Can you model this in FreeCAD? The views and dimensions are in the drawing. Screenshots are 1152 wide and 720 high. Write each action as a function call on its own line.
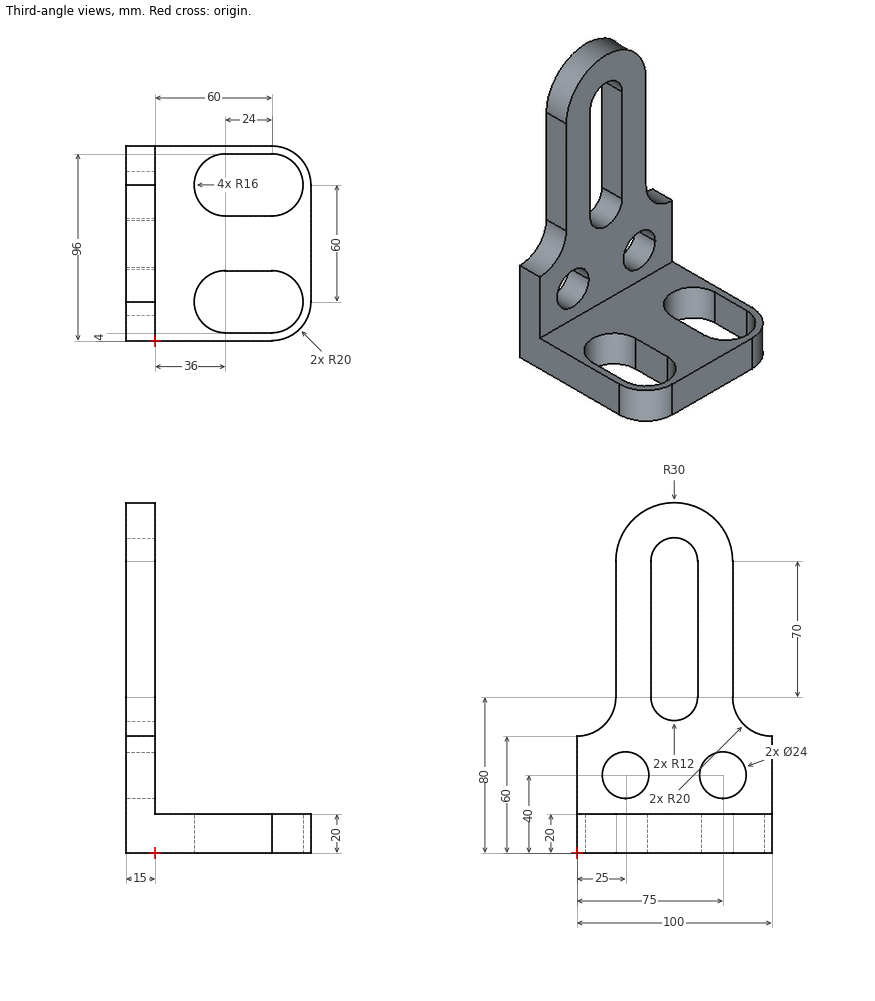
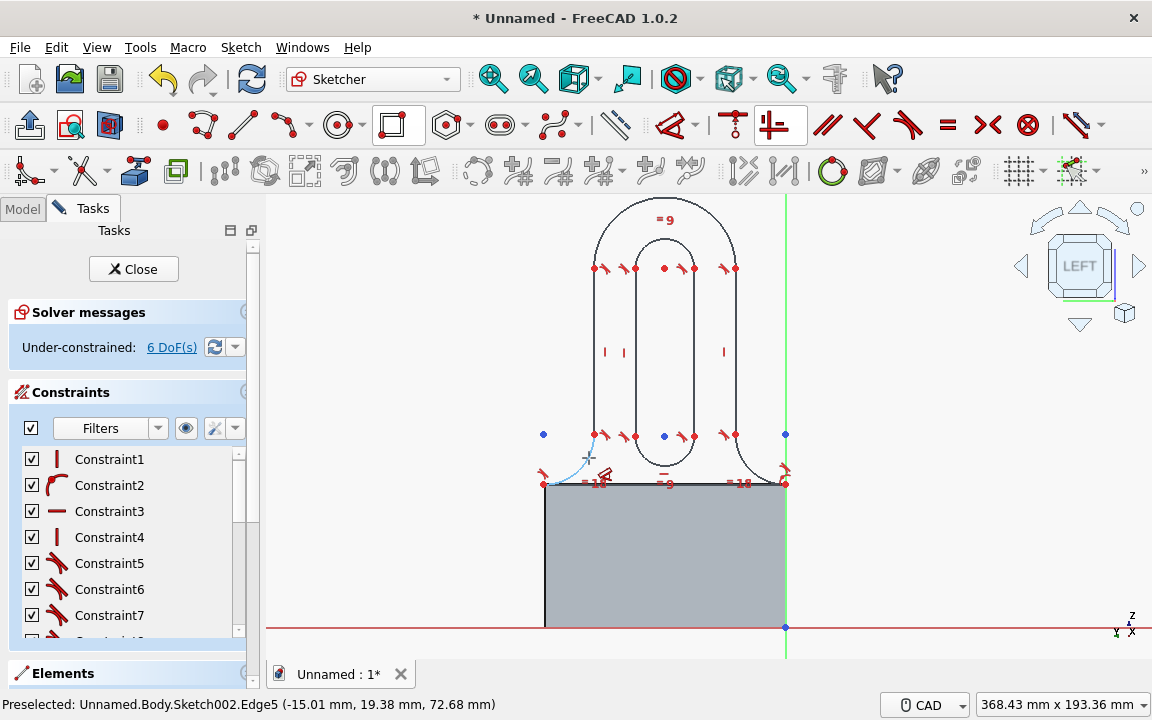
click(589, 457)
click(618, 471)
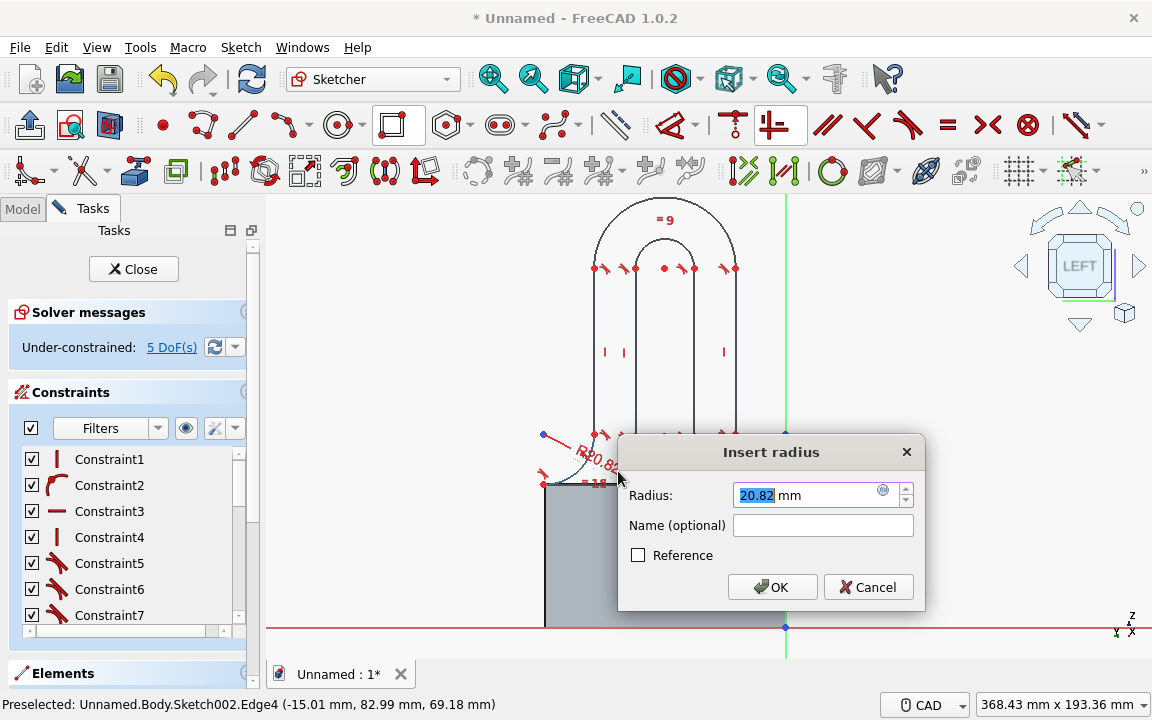
text(20)
key(Return)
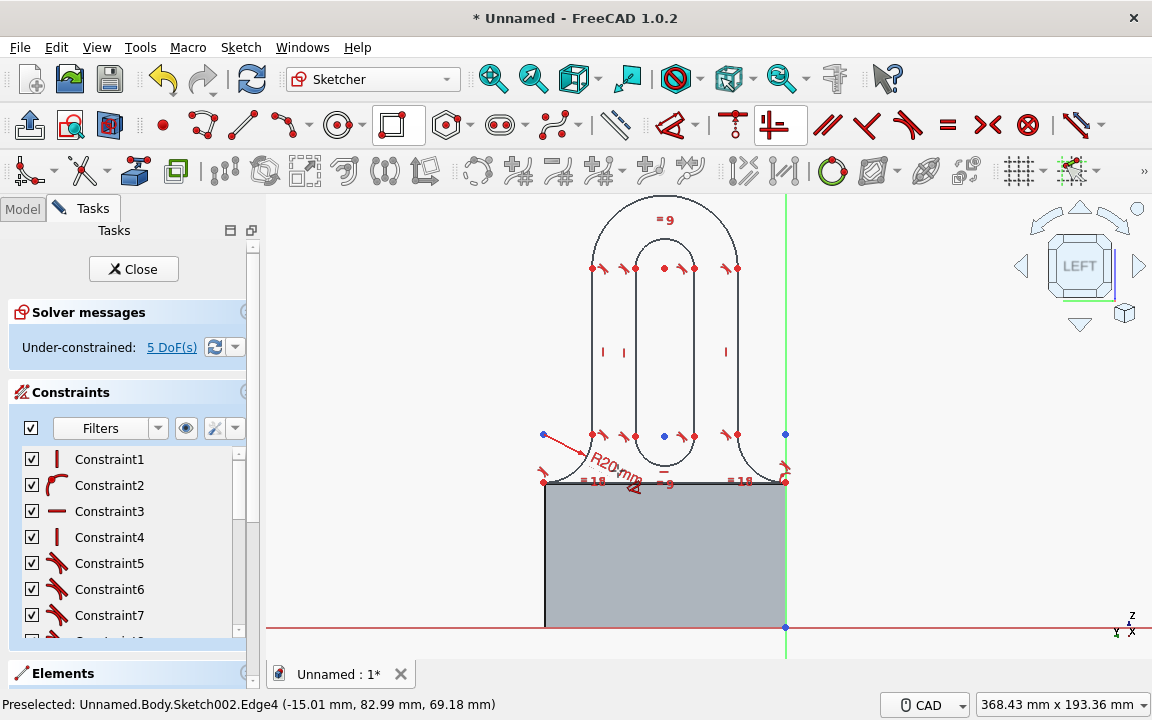
click(724, 226)
click(769, 256)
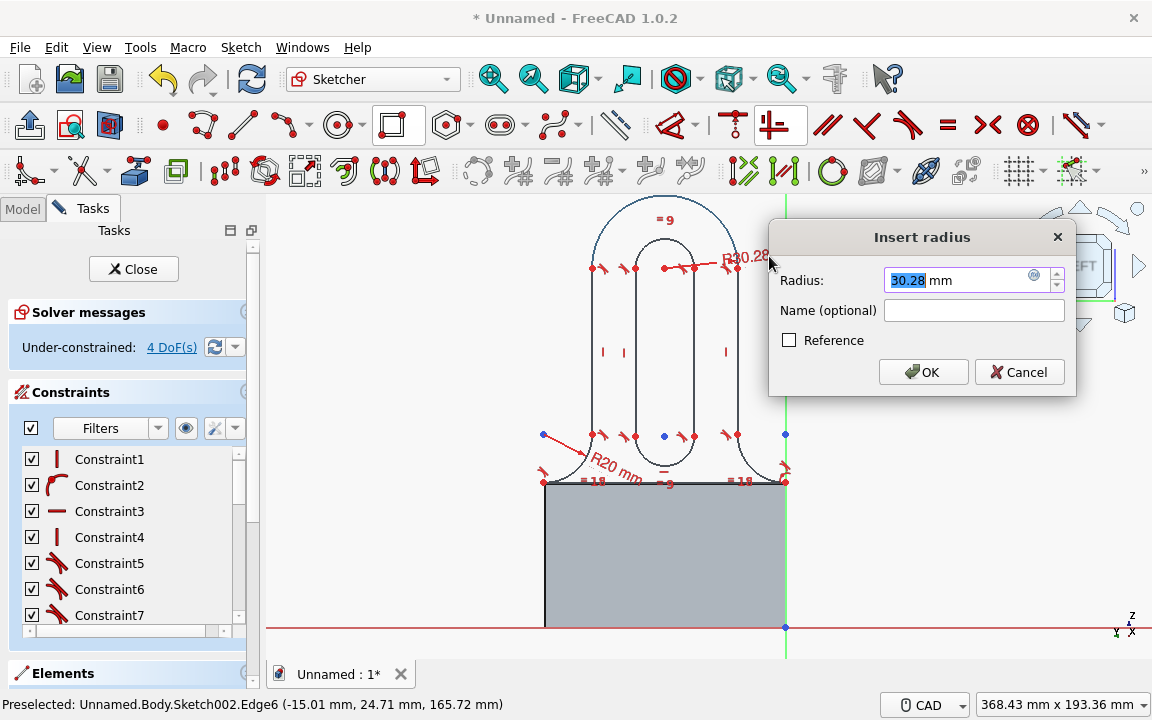
text(30)
key(Return)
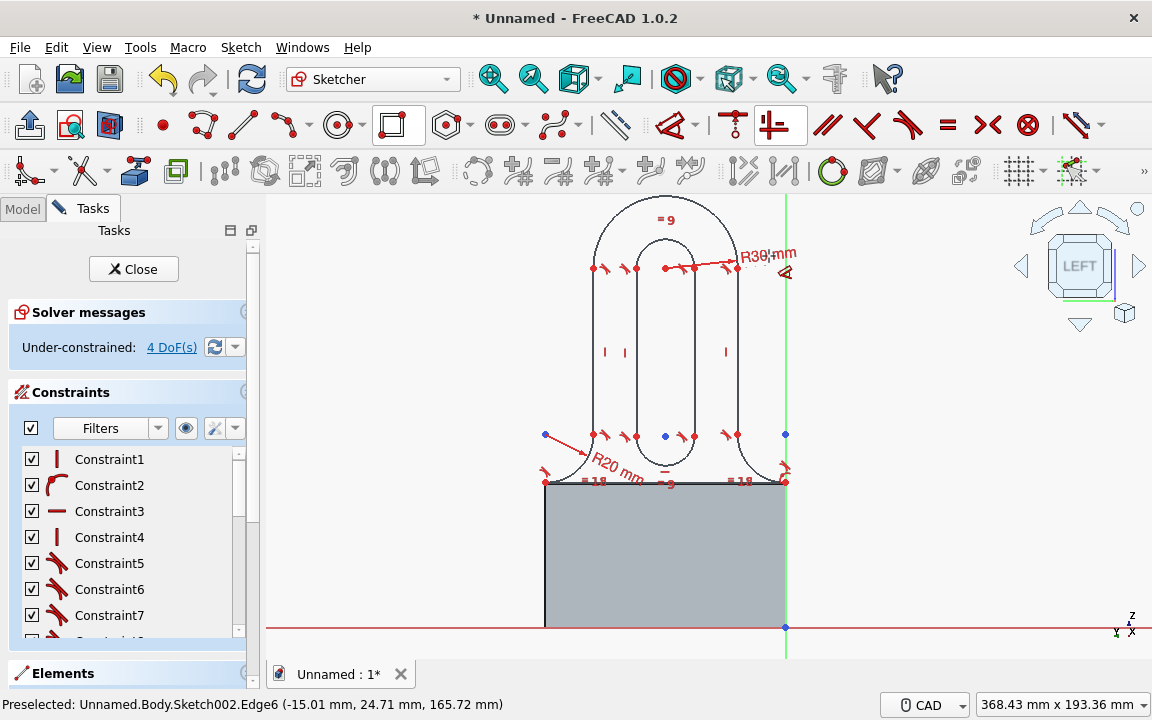
scroll(649, 460, up, 2)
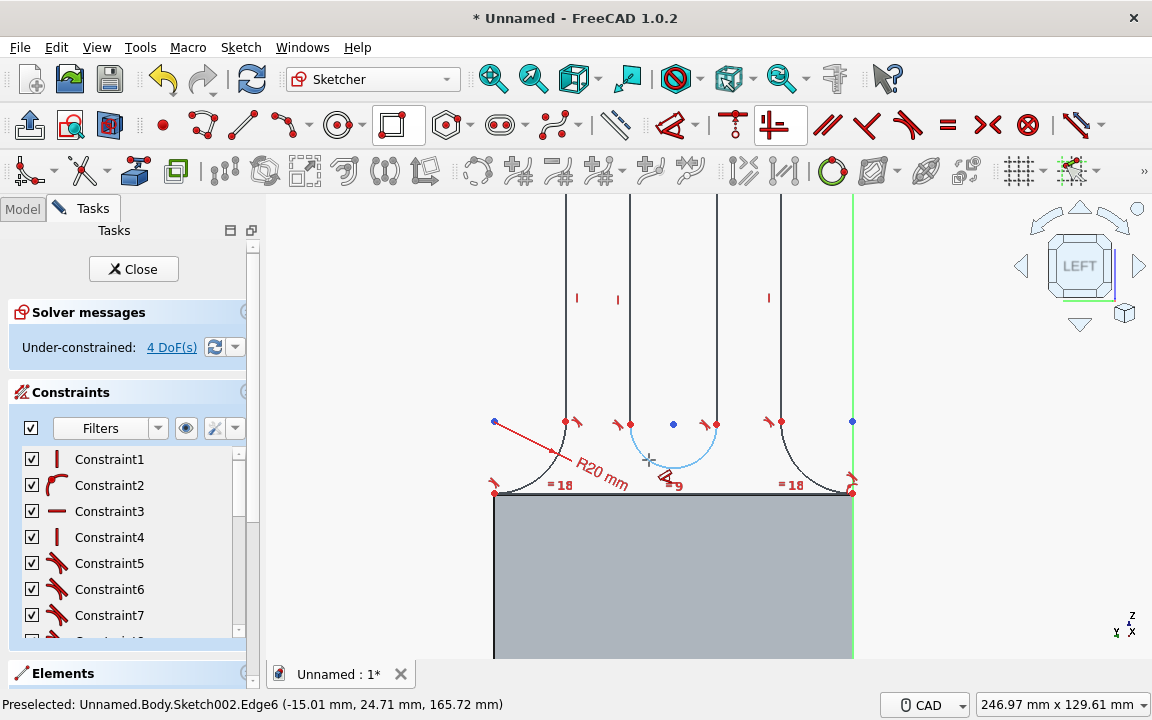
click(648, 460)
click(598, 421)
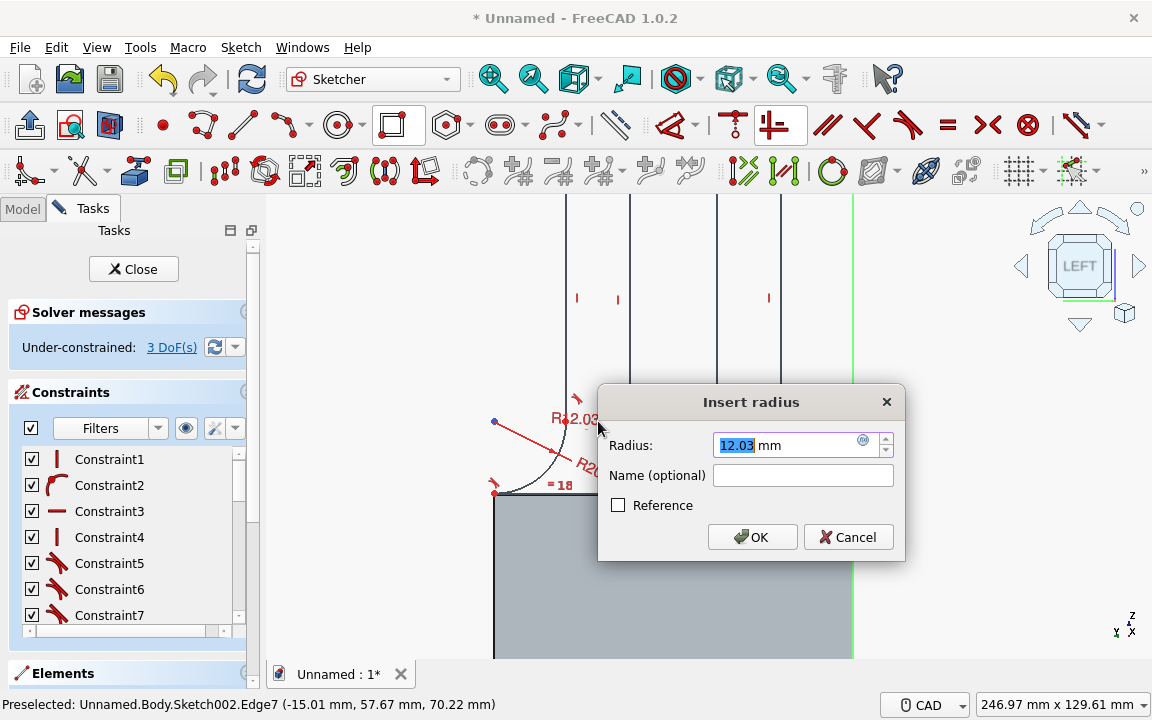
text(12)
key(Return)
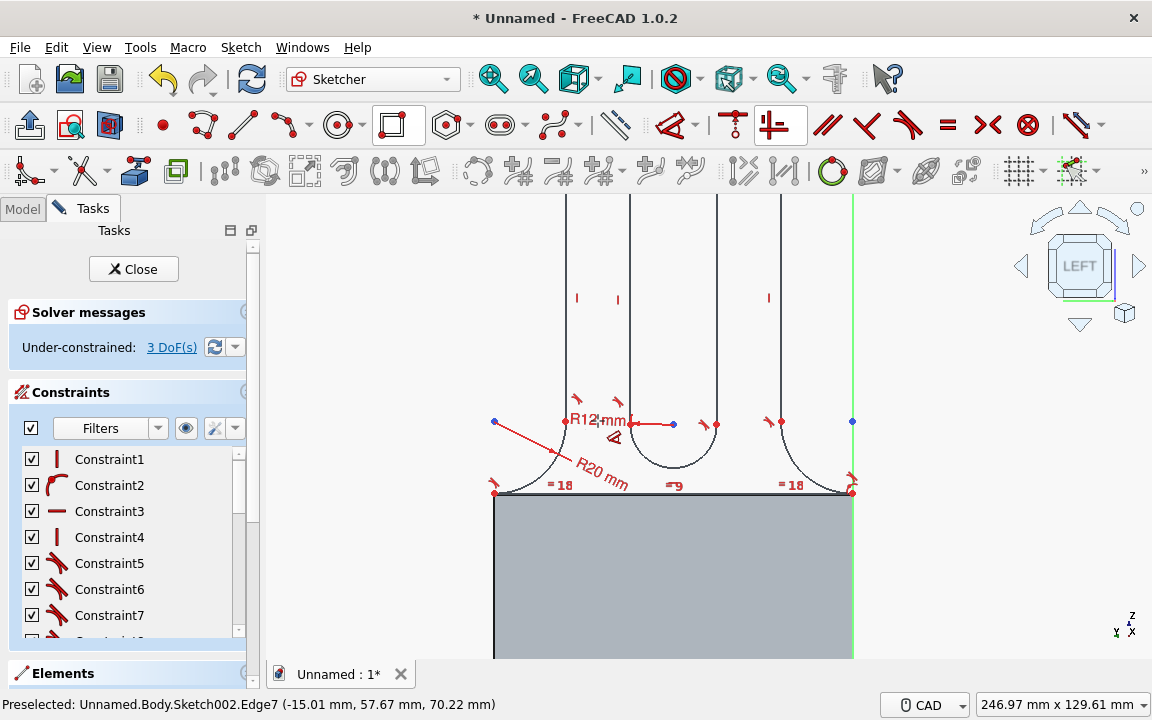
click(566, 248)
click(532, 322)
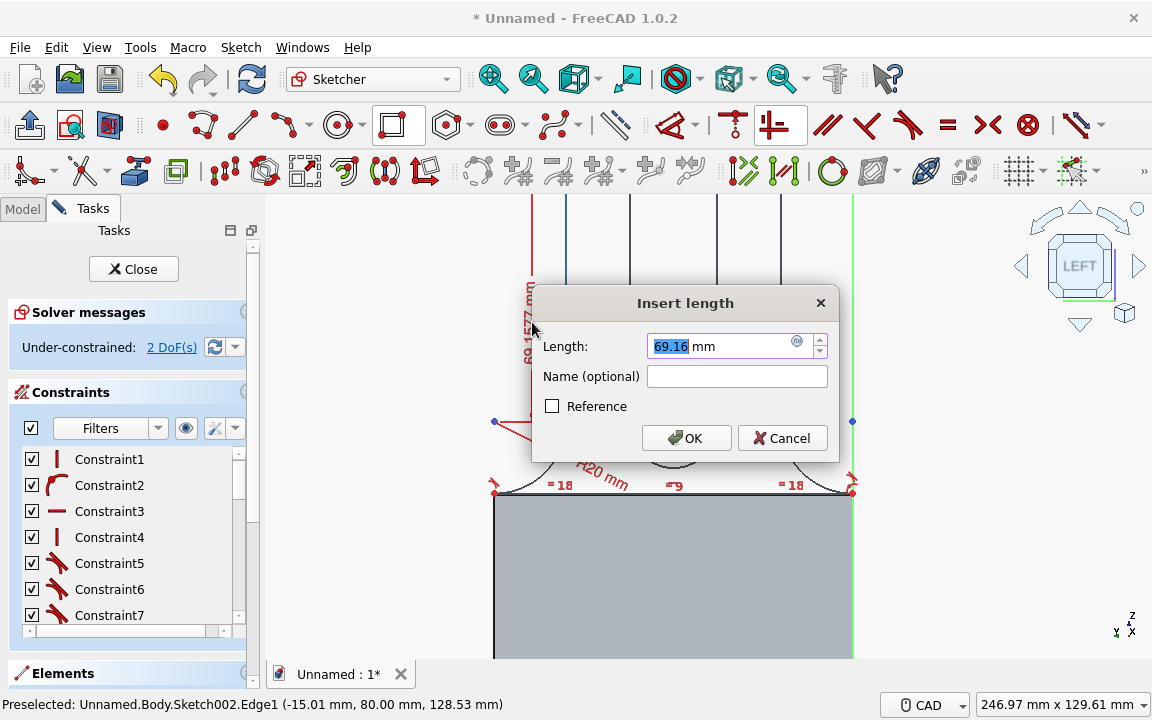
text(70)
key(Return)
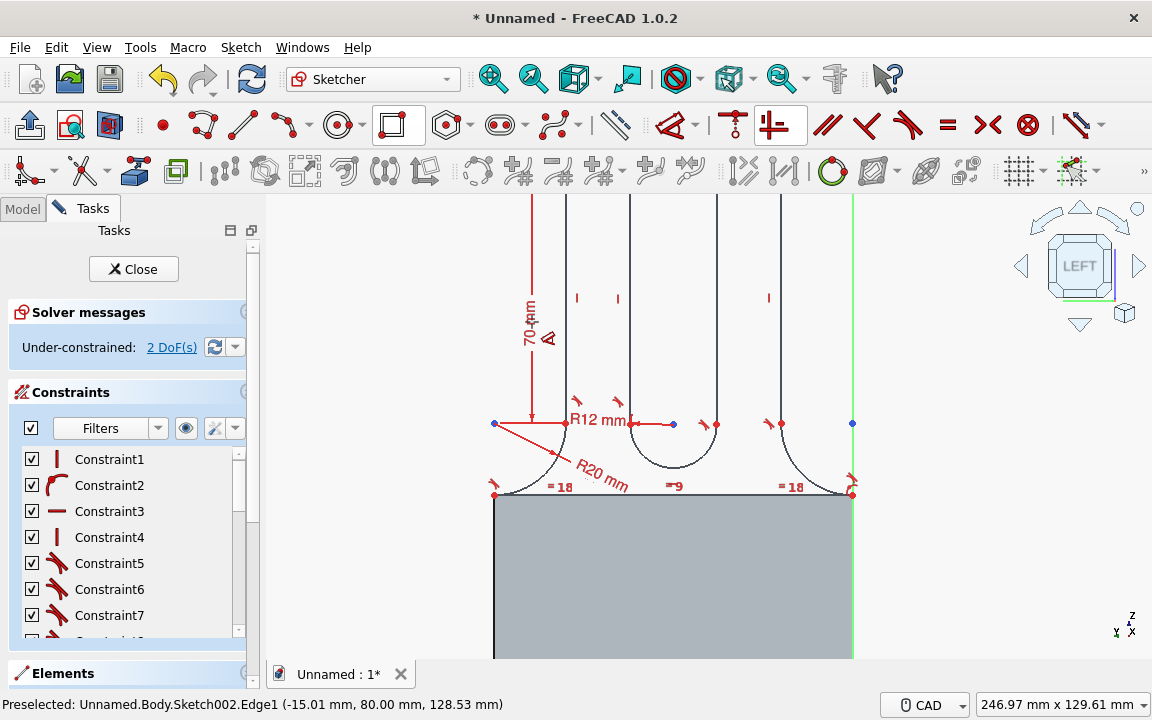
click(630, 349)
click(596, 277)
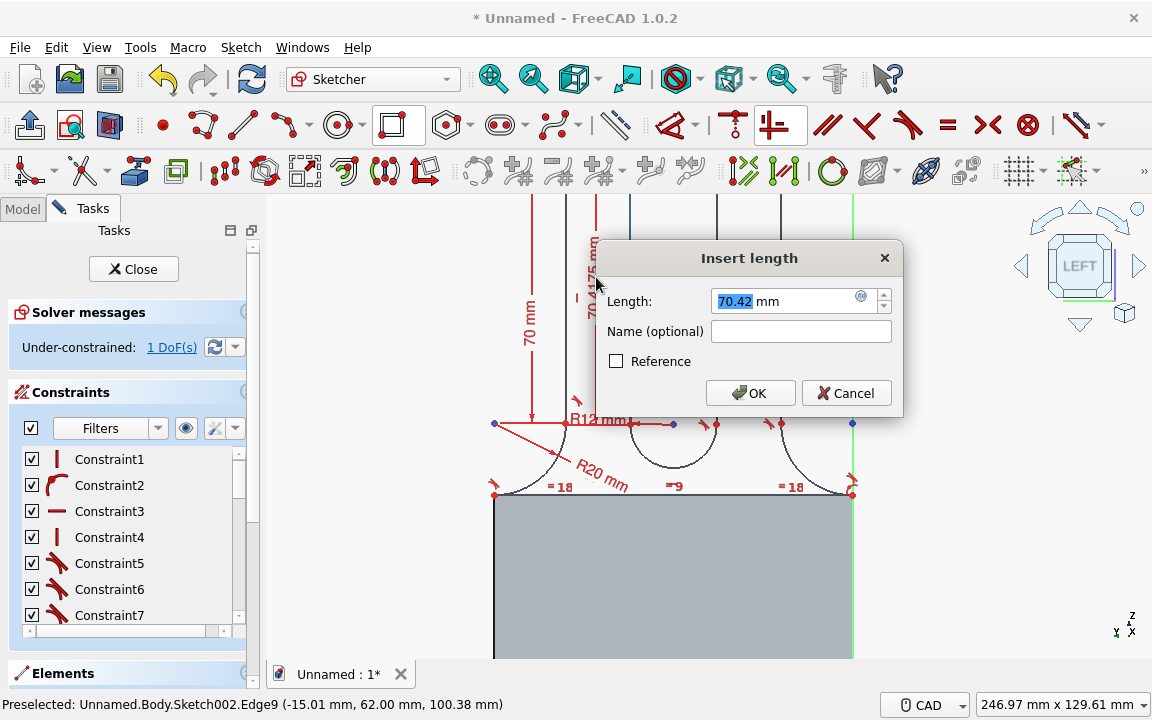
text(70)
key(Return)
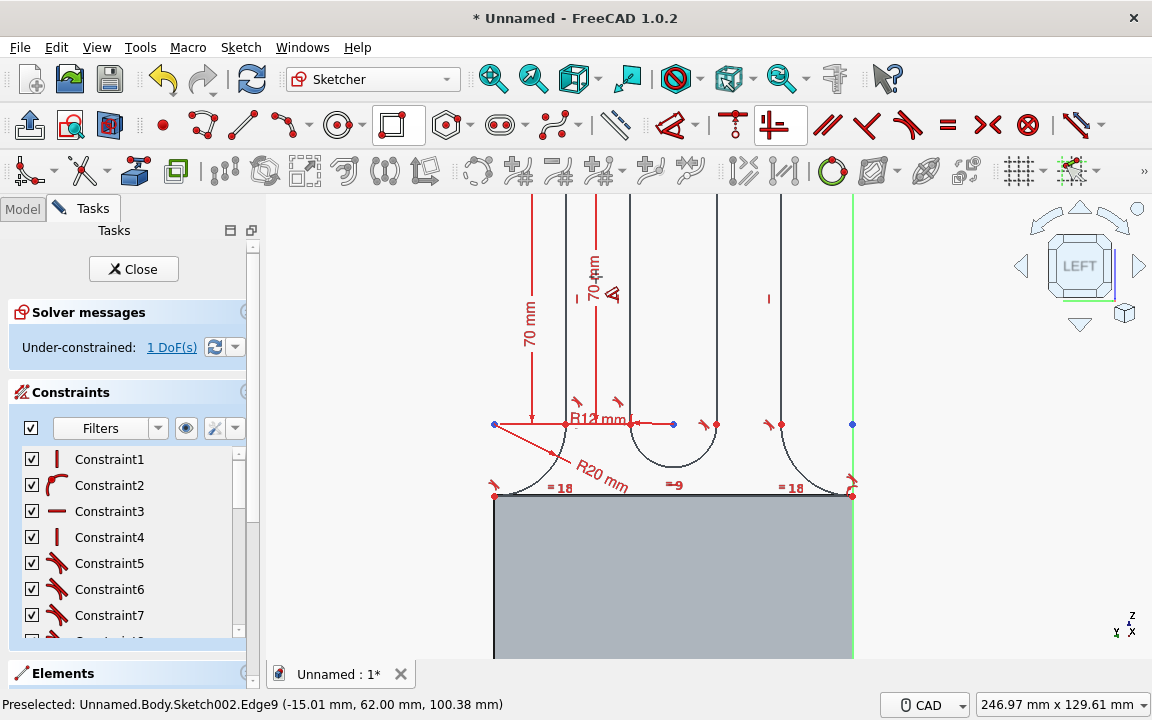
click(566, 424)
click(887, 528)